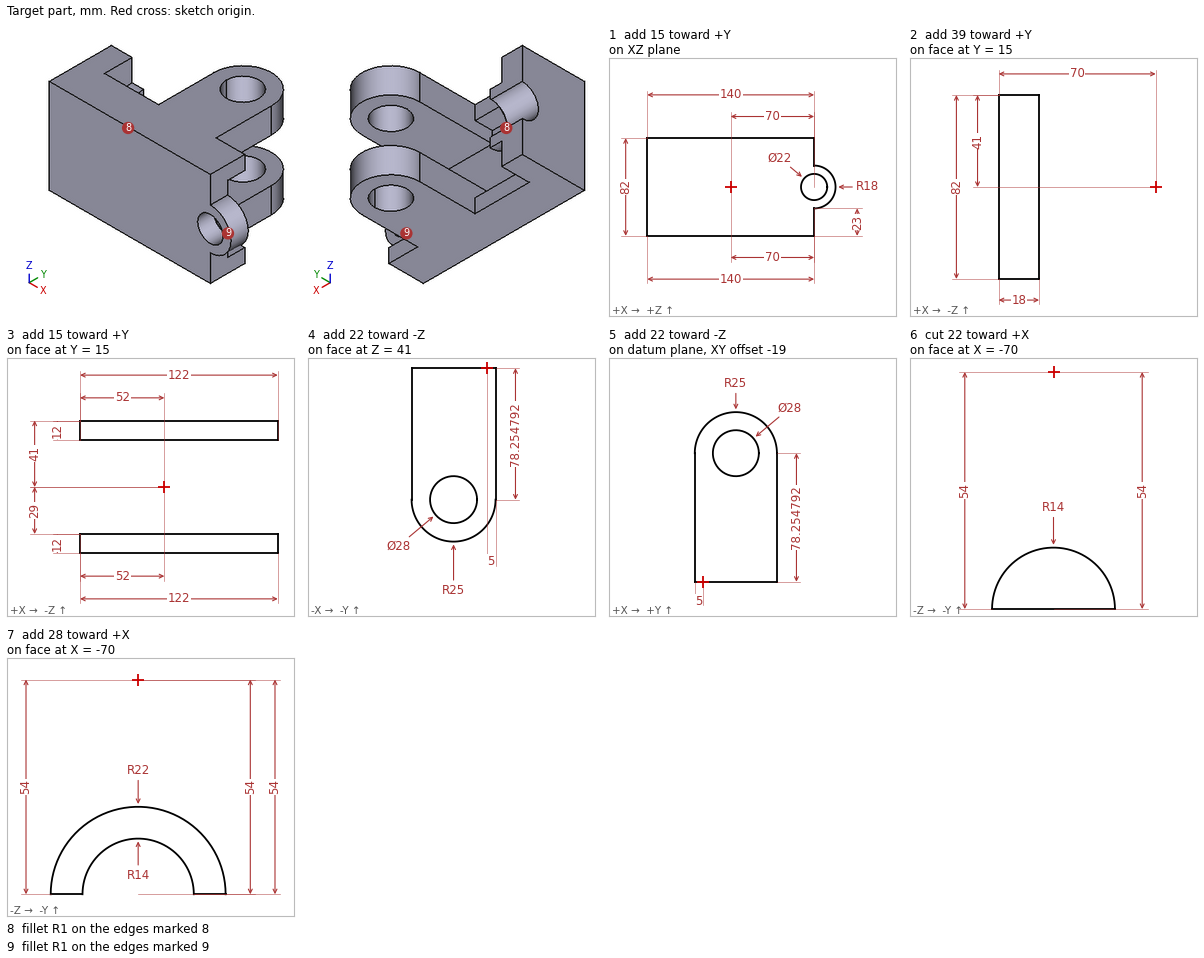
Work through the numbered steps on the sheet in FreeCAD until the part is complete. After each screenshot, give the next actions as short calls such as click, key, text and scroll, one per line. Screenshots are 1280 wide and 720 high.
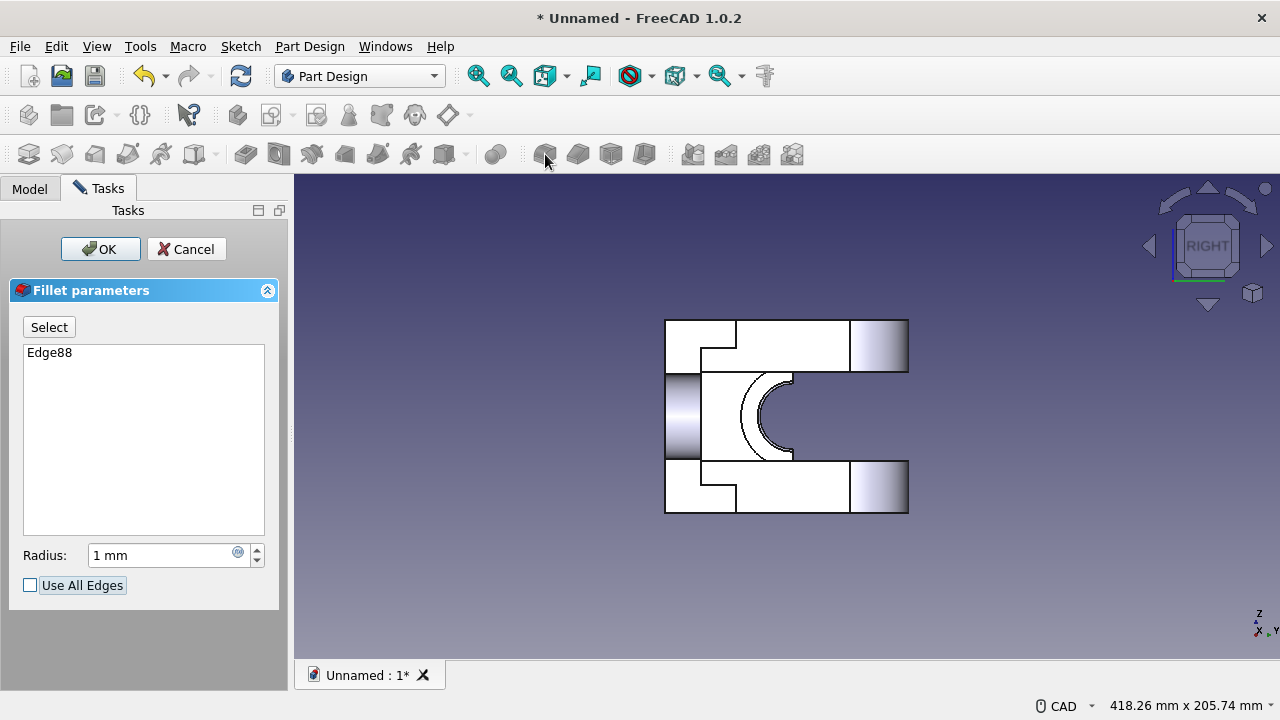
click(101, 249)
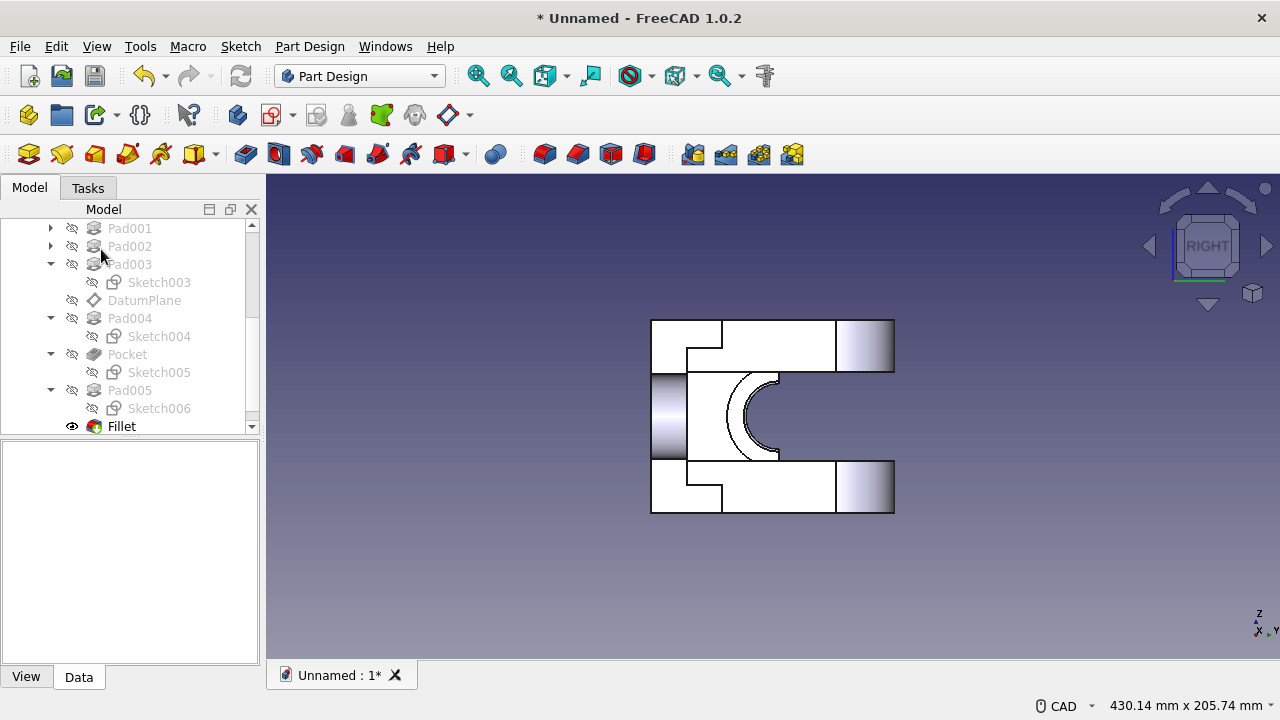
click(479, 76)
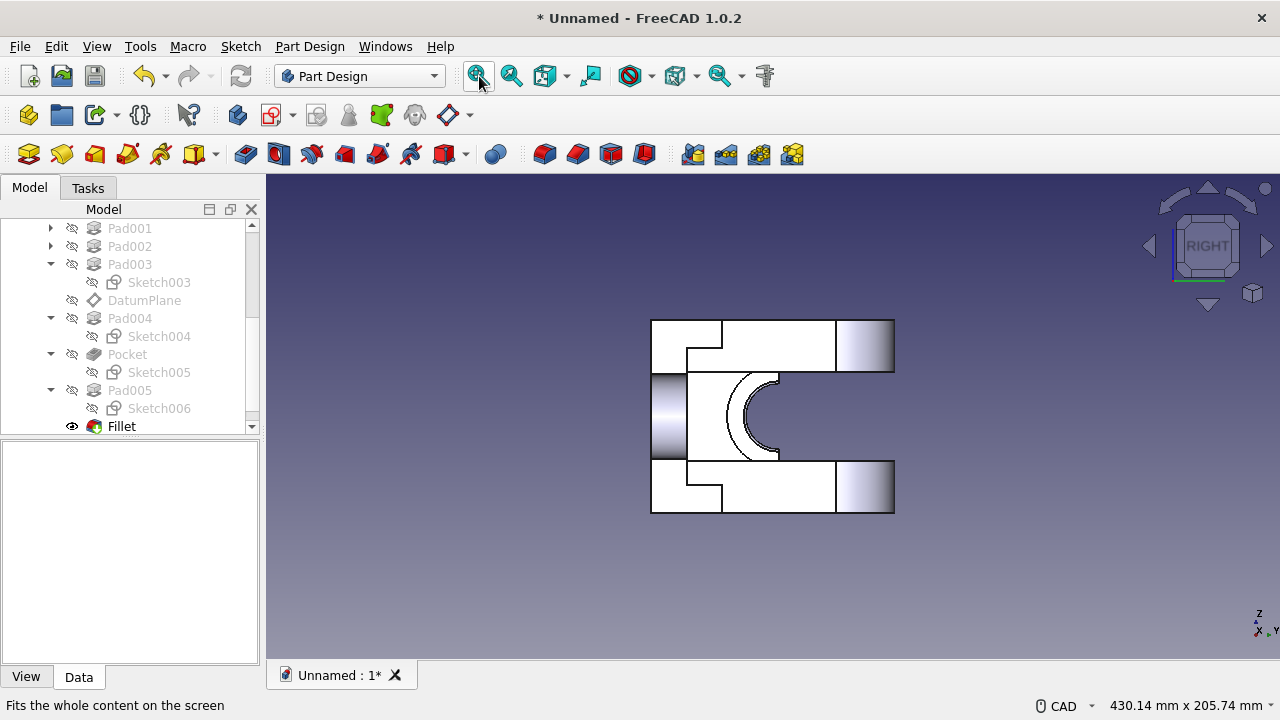
key(0)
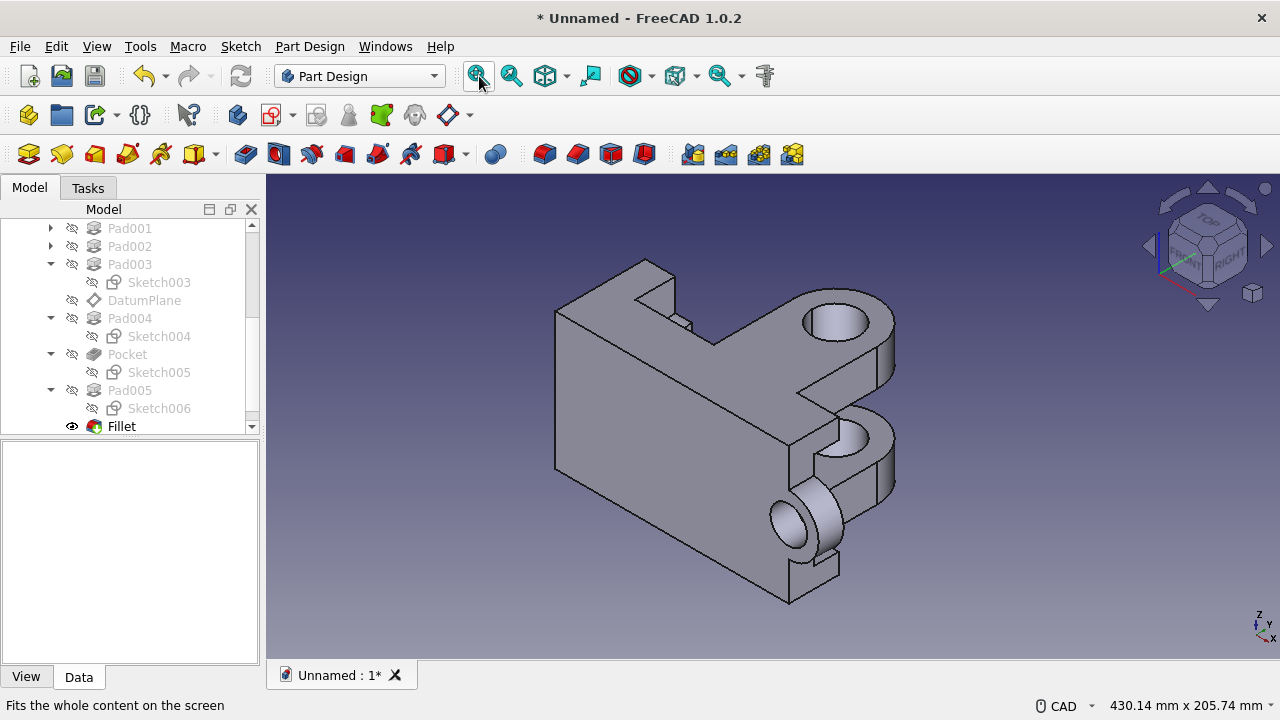
key(2)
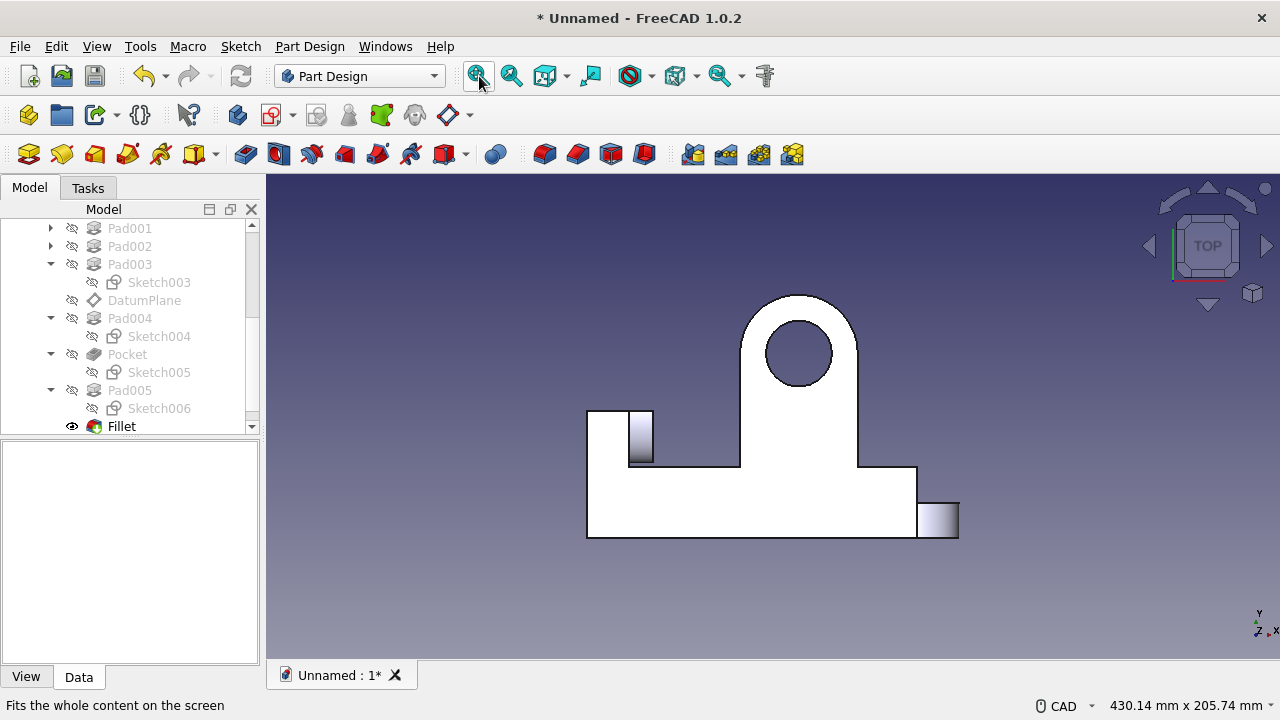
key(1)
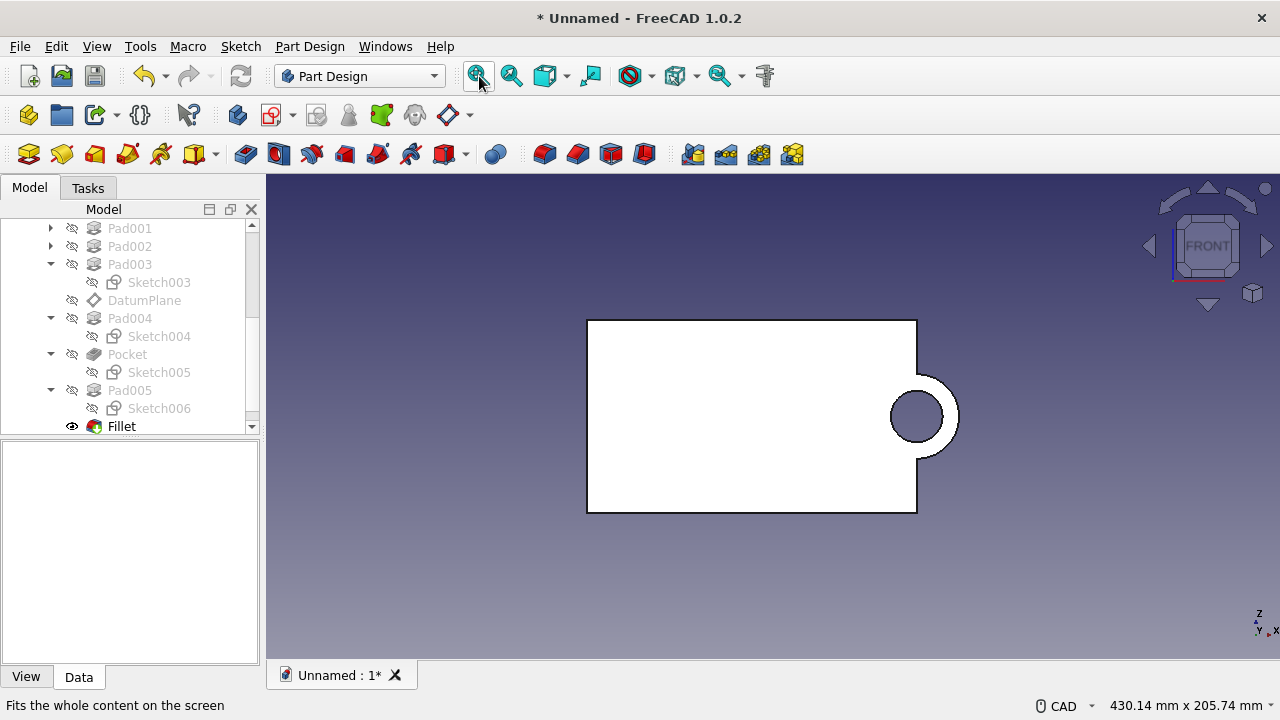
click(479, 76)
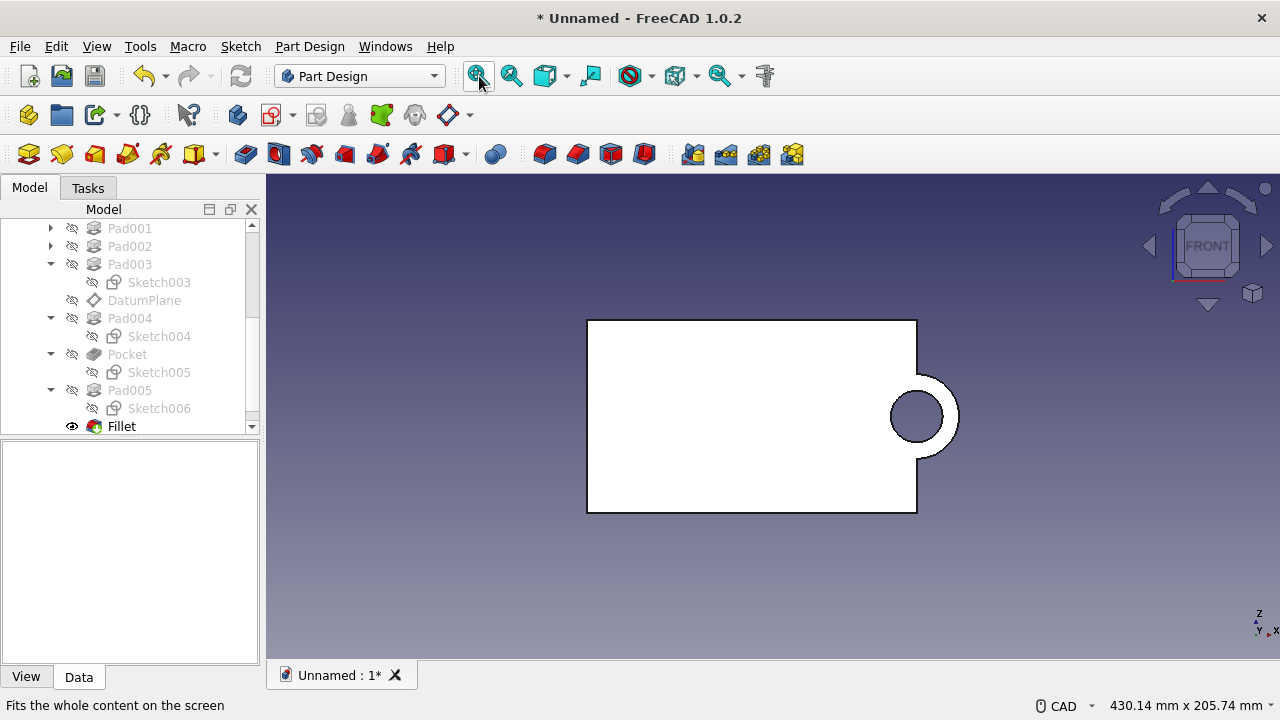
key(3)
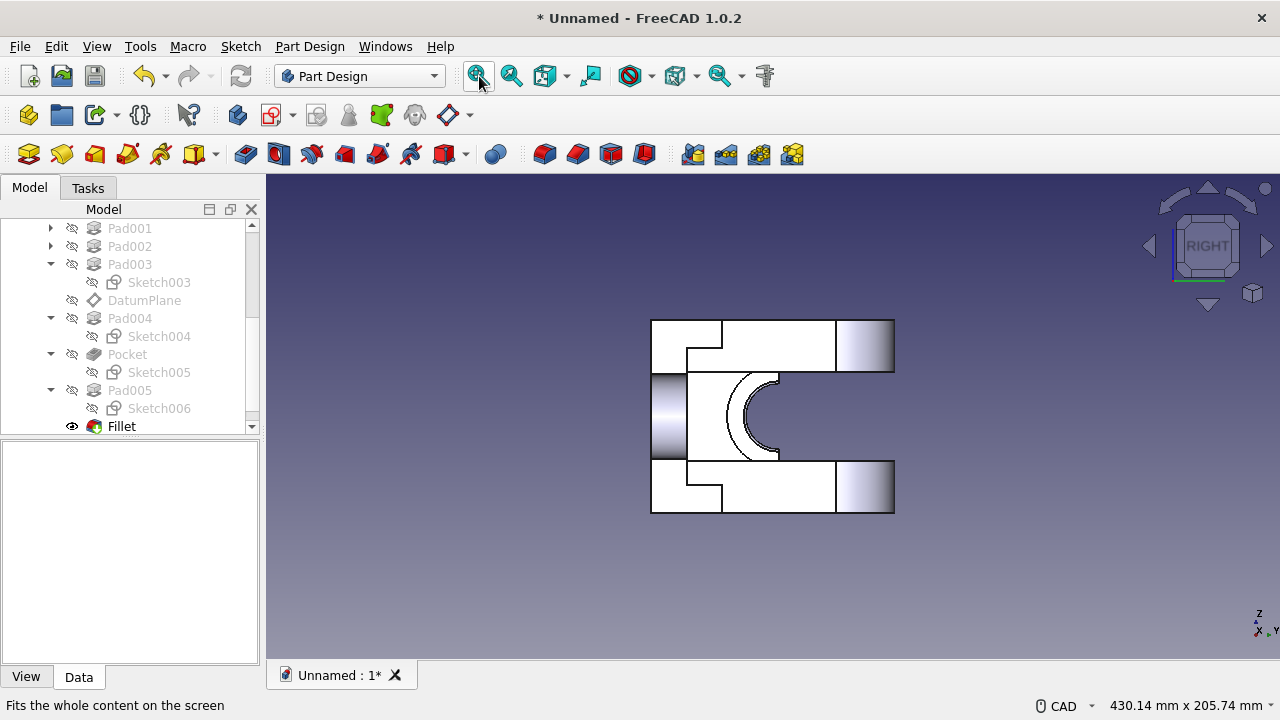
click(479, 76)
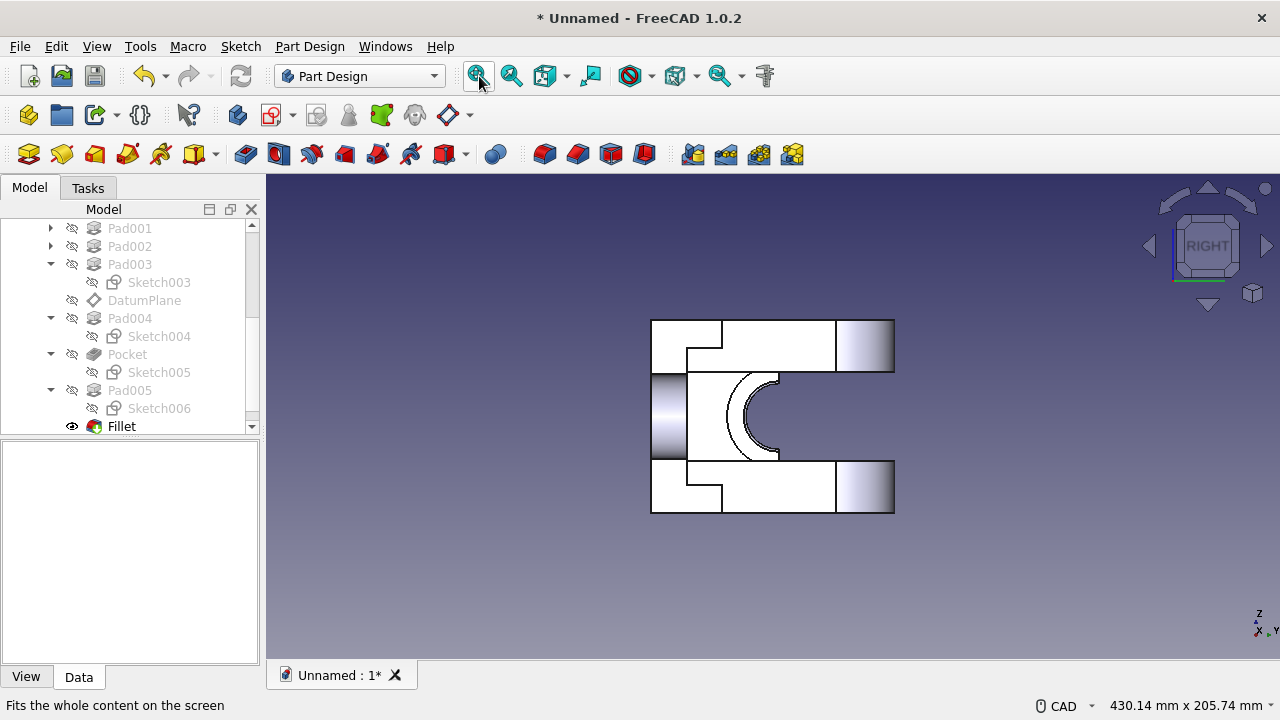
key(5)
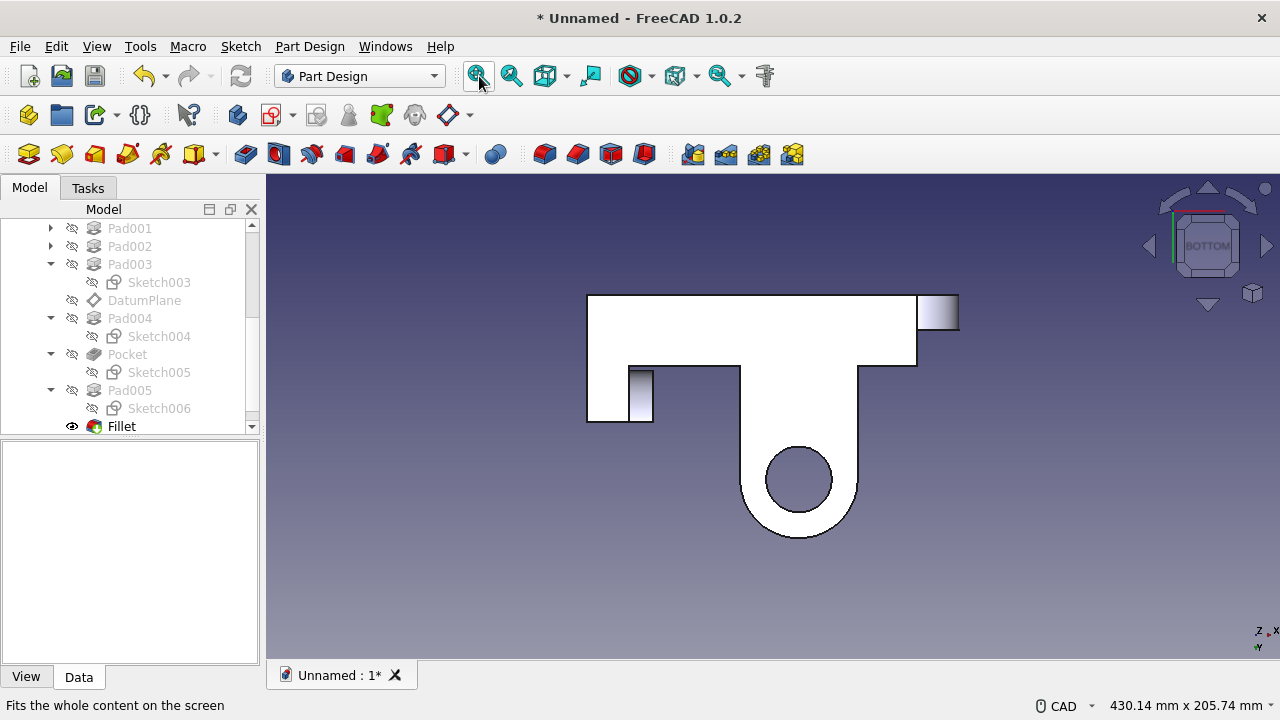
key(4)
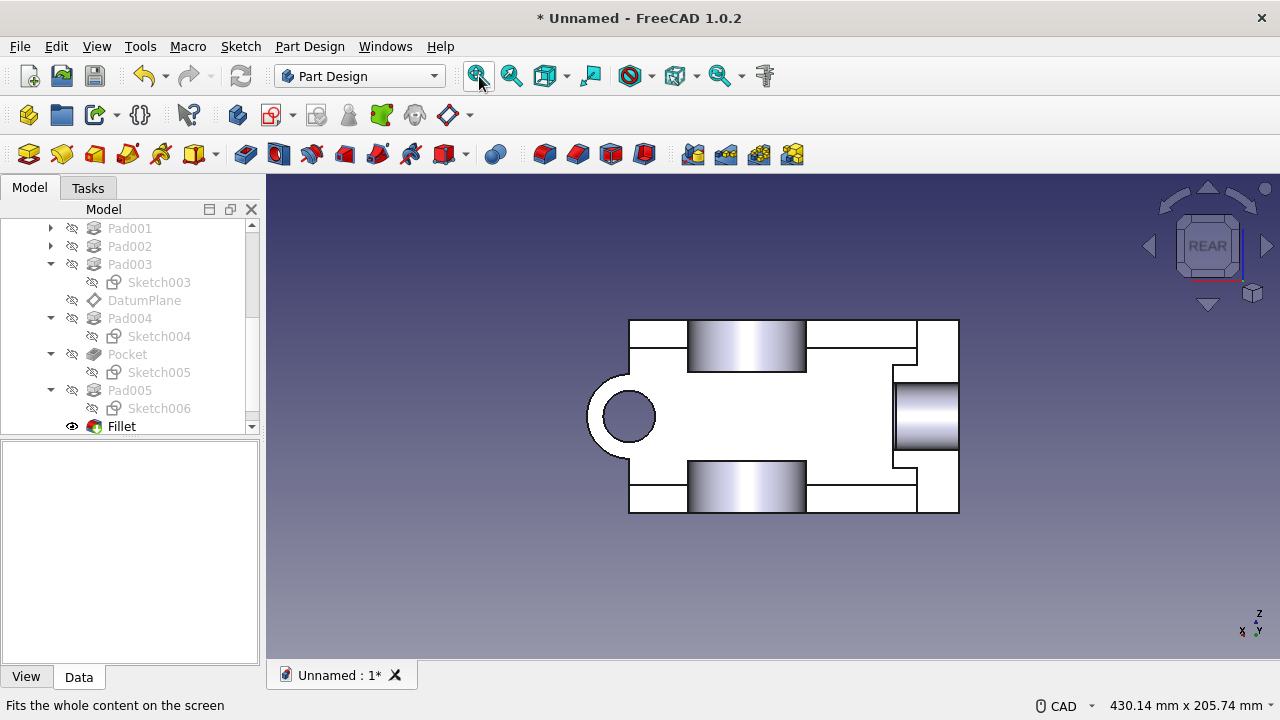
click(479, 76)